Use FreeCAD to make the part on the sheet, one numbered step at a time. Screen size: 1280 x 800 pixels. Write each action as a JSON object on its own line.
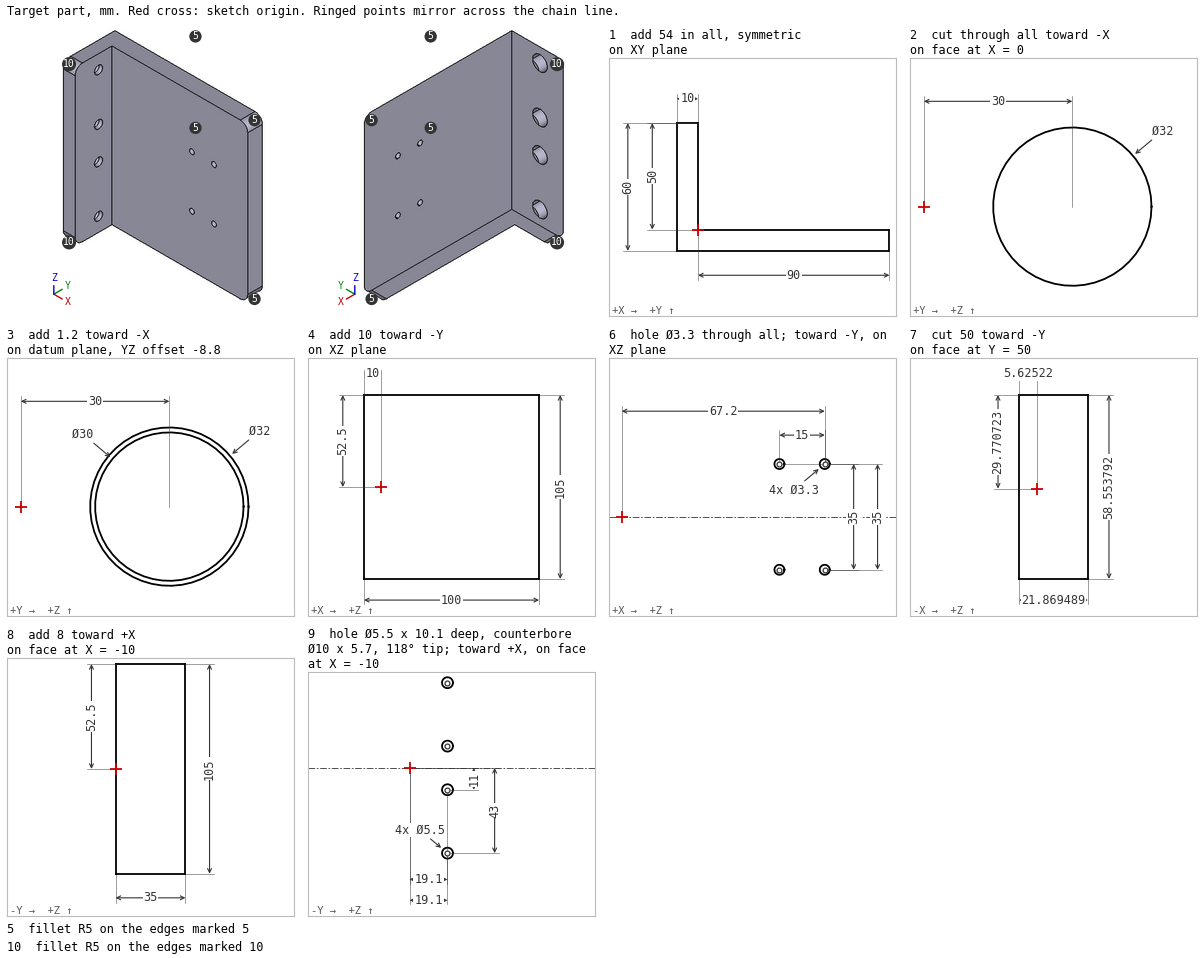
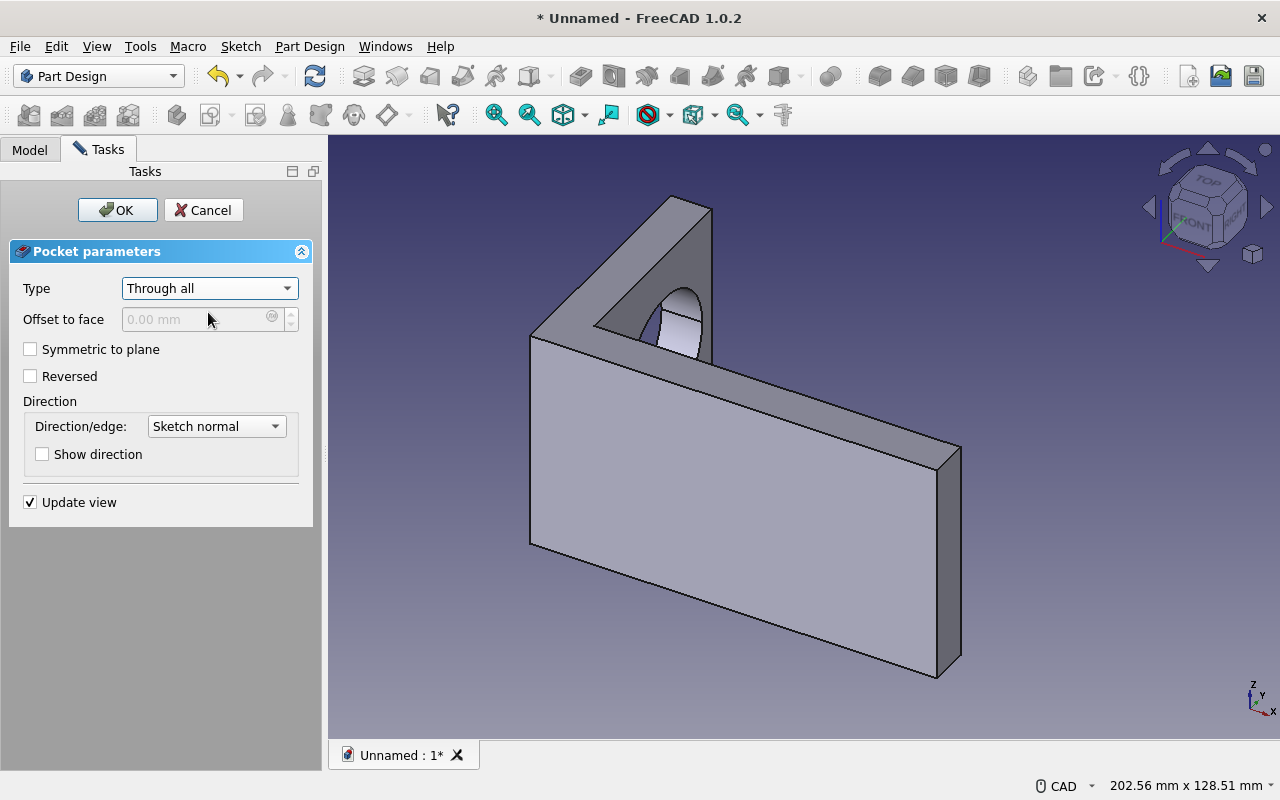
{"action": "left_click", "coordinate": [118, 210]}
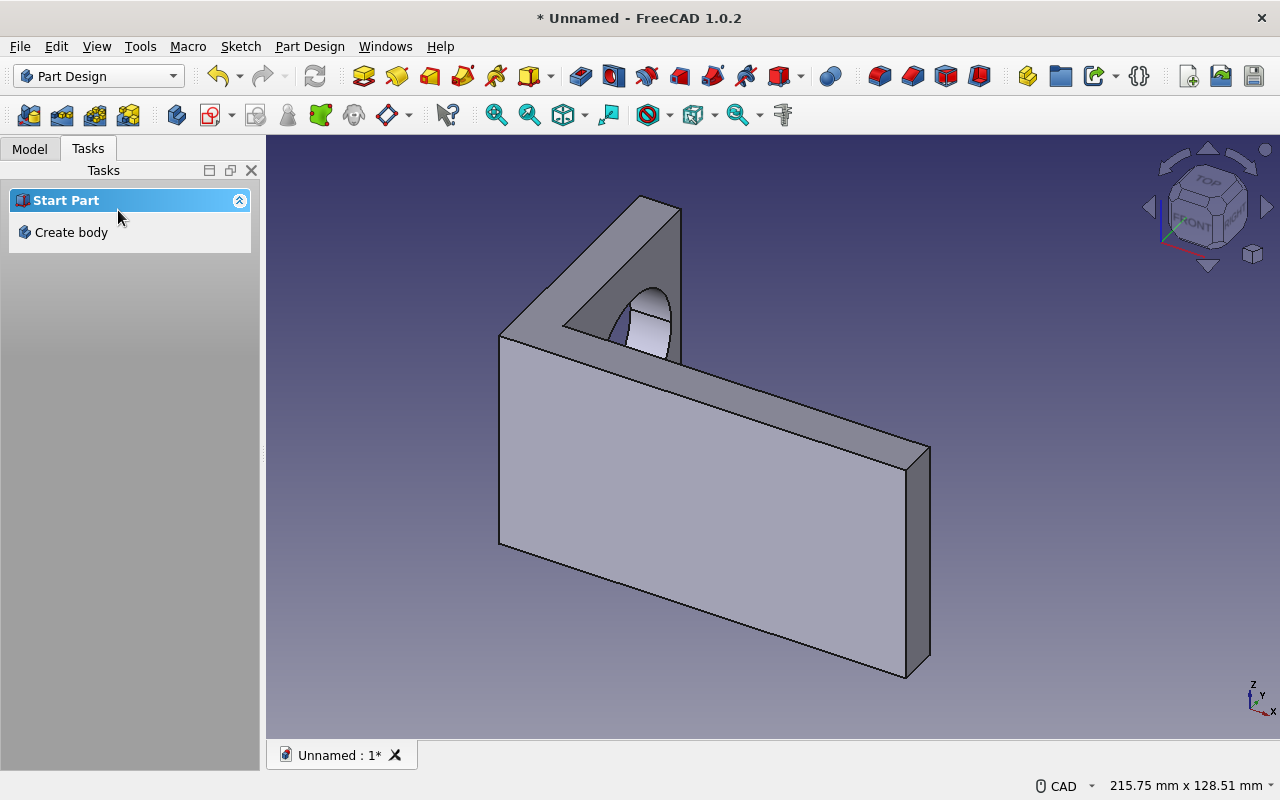
{"action": "left_click", "coordinate": [30, 148]}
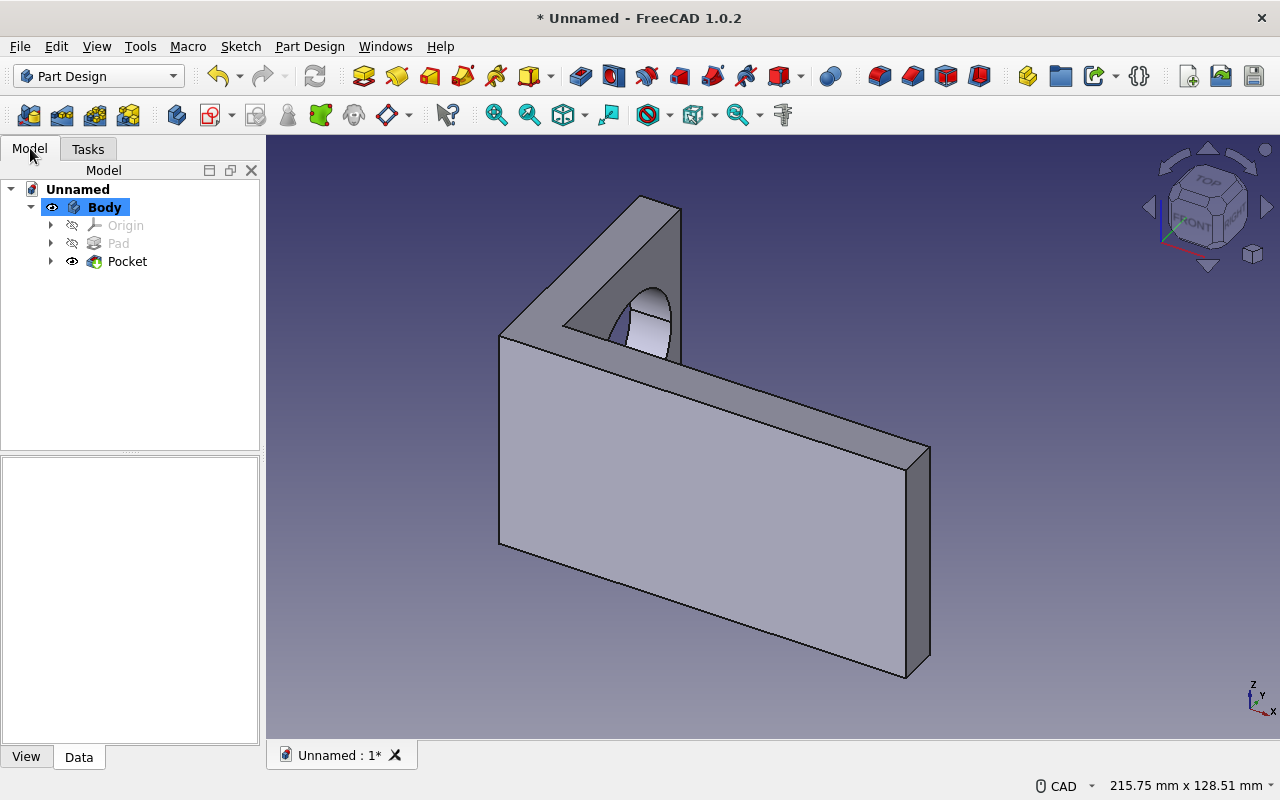
{"action": "left_click", "coordinate": [51, 225]}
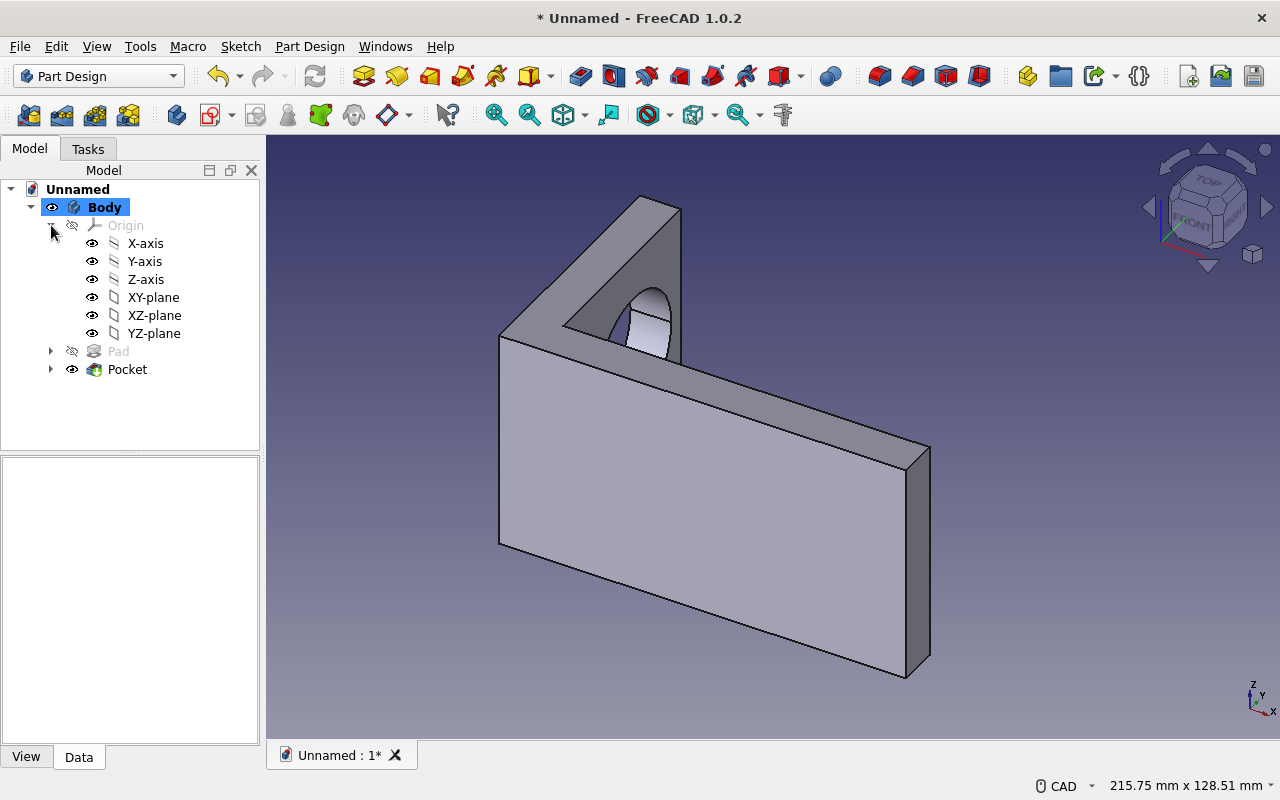
{"action": "left_click", "coordinate": [137, 333]}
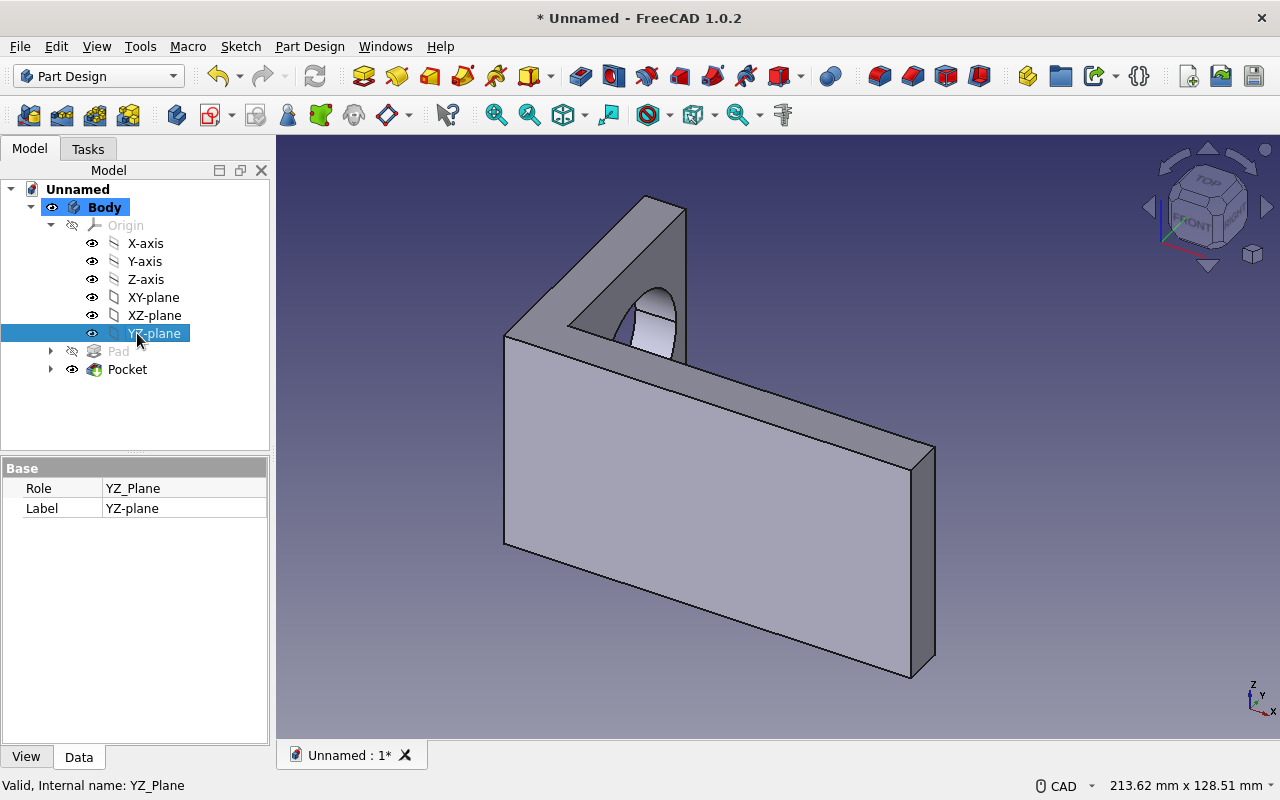
{"action": "left_click", "coordinate": [386, 116]}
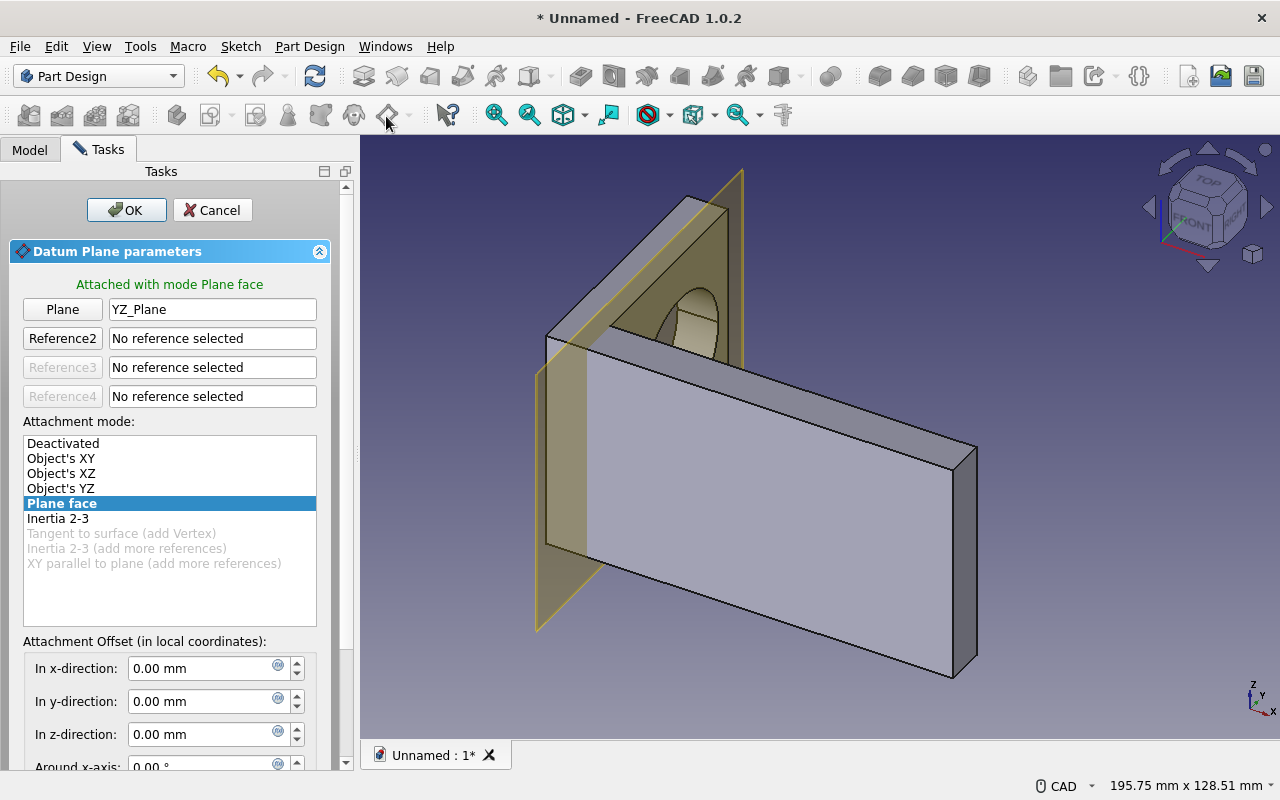
{"action": "triple_click", "coordinate": [210, 734]}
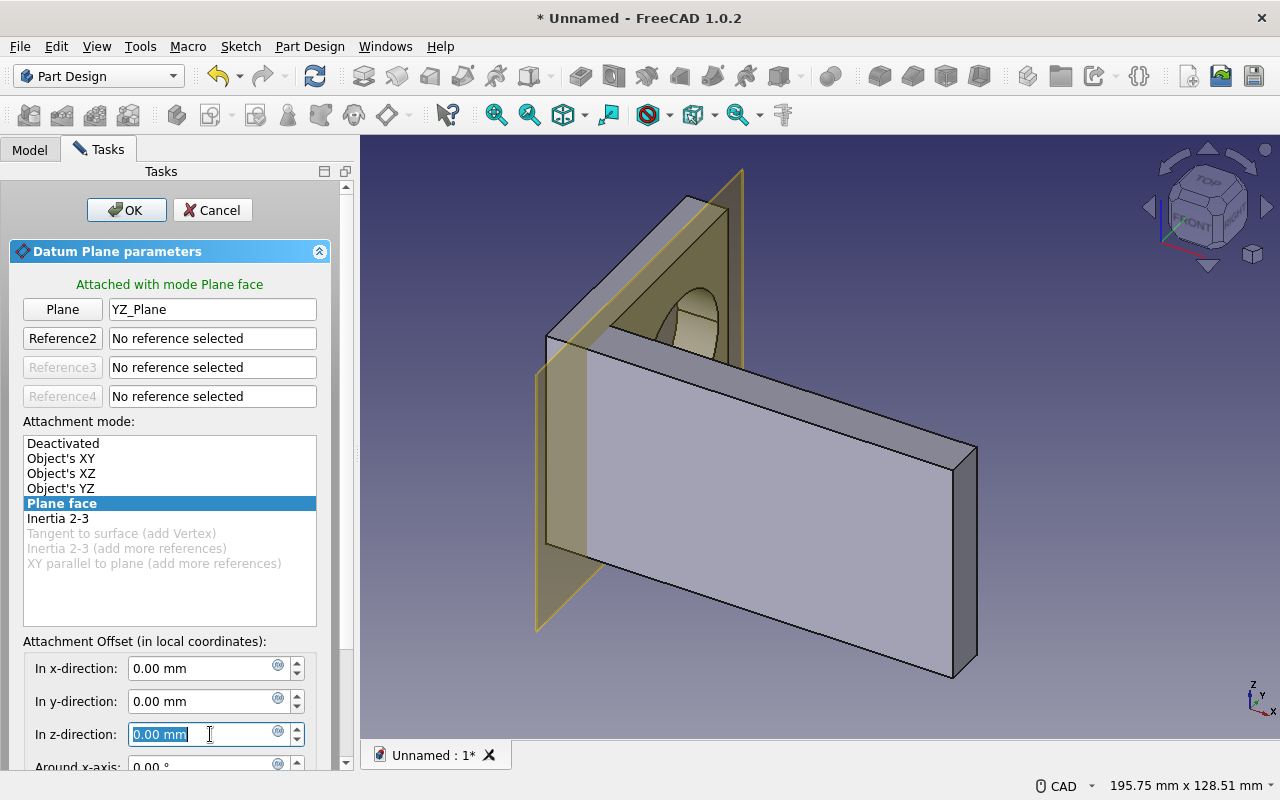
{"action": "type", "text": "-8.8"}
{"action": "key", "text": "Tab"}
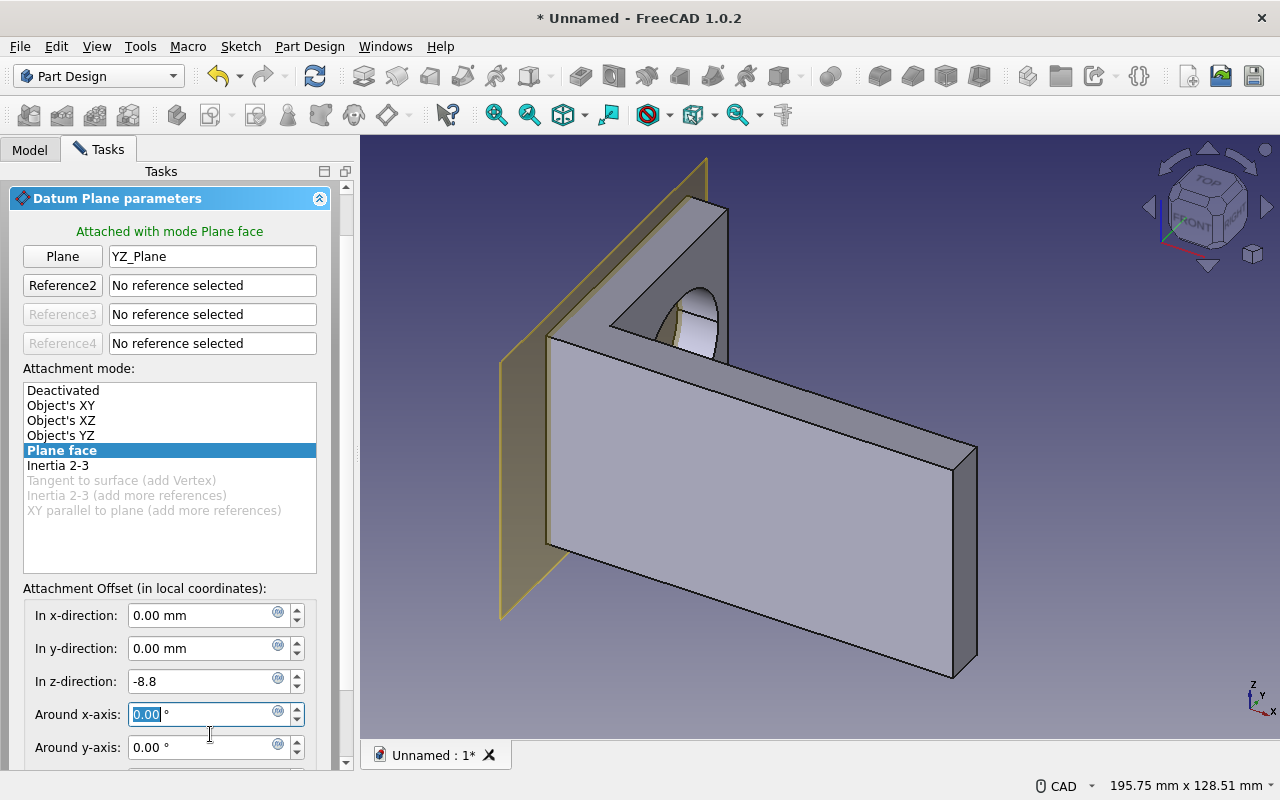
{"action": "scroll", "coordinate": [346, 476], "scroll_direction": "up", "scroll_amount": 2}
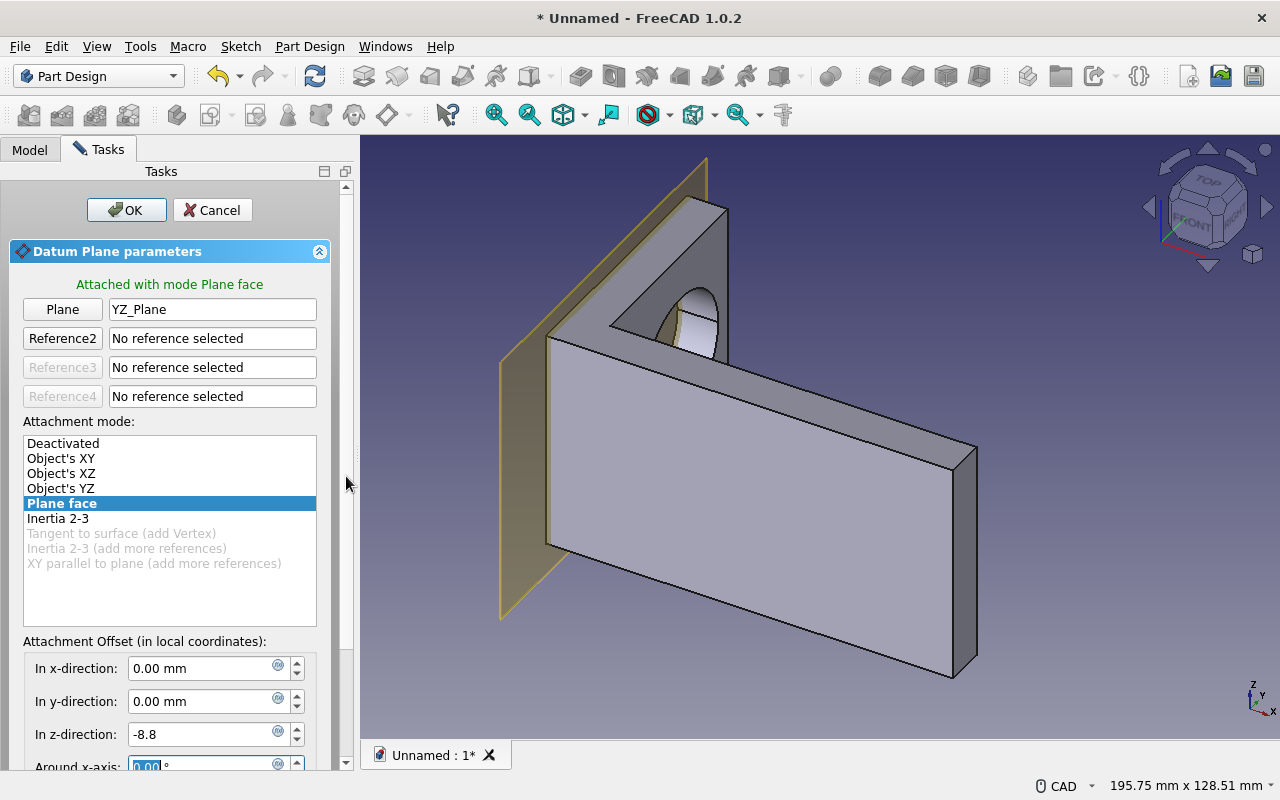
{"action": "left_click", "coordinate": [127, 210]}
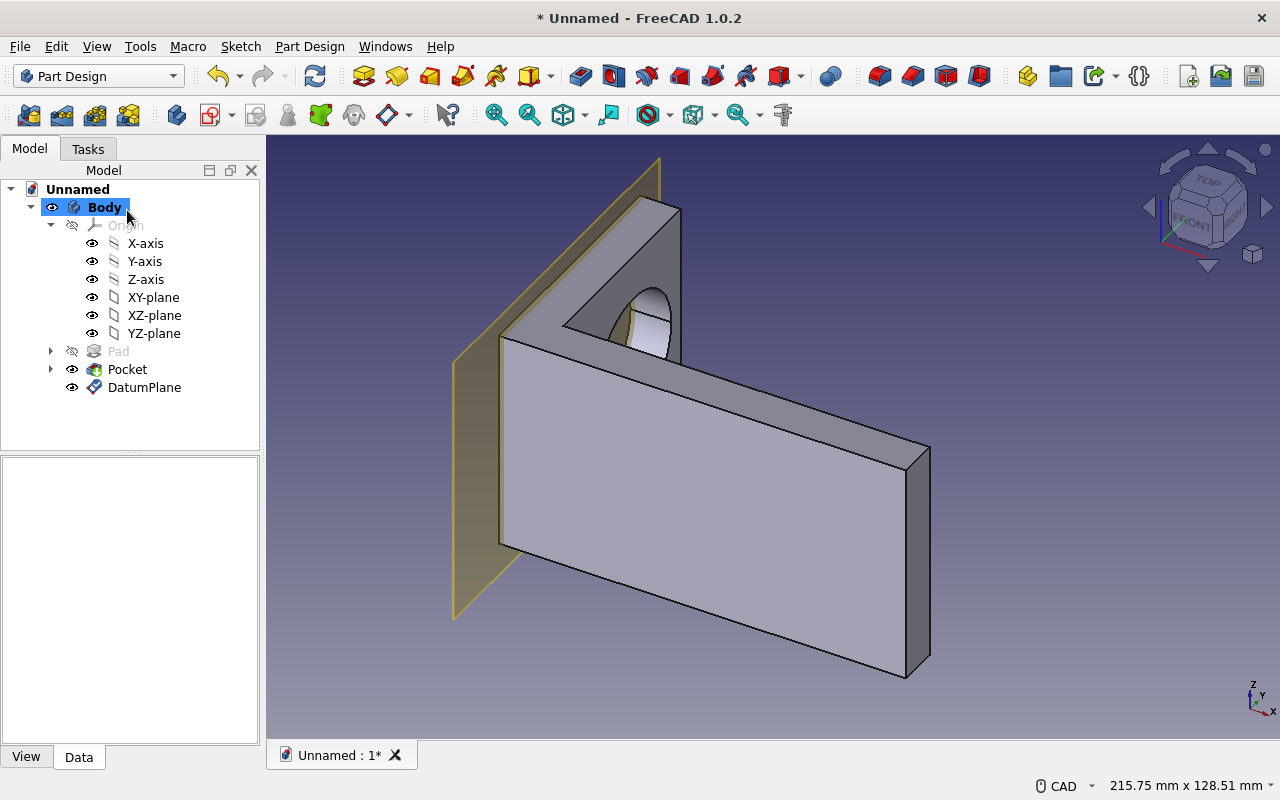
{"action": "left_click", "coordinate": [117, 387]}